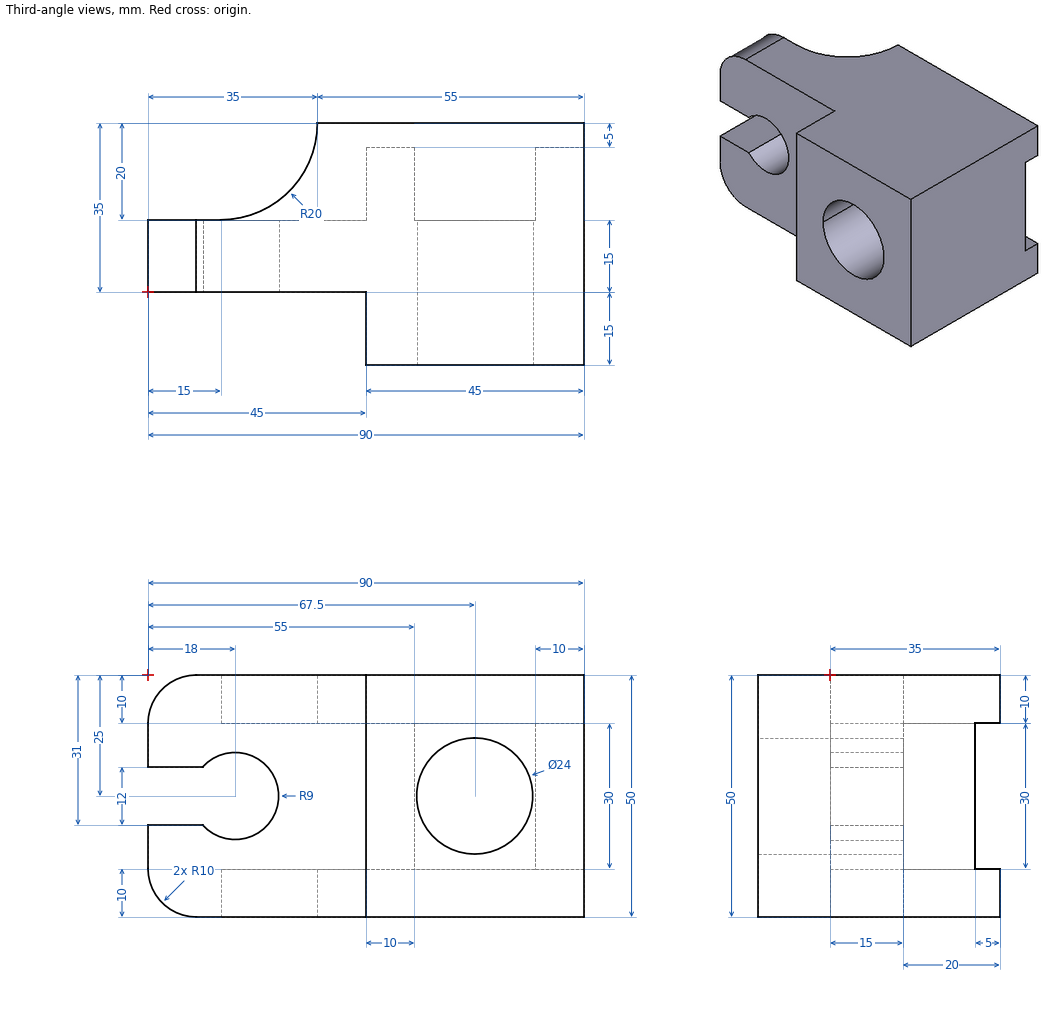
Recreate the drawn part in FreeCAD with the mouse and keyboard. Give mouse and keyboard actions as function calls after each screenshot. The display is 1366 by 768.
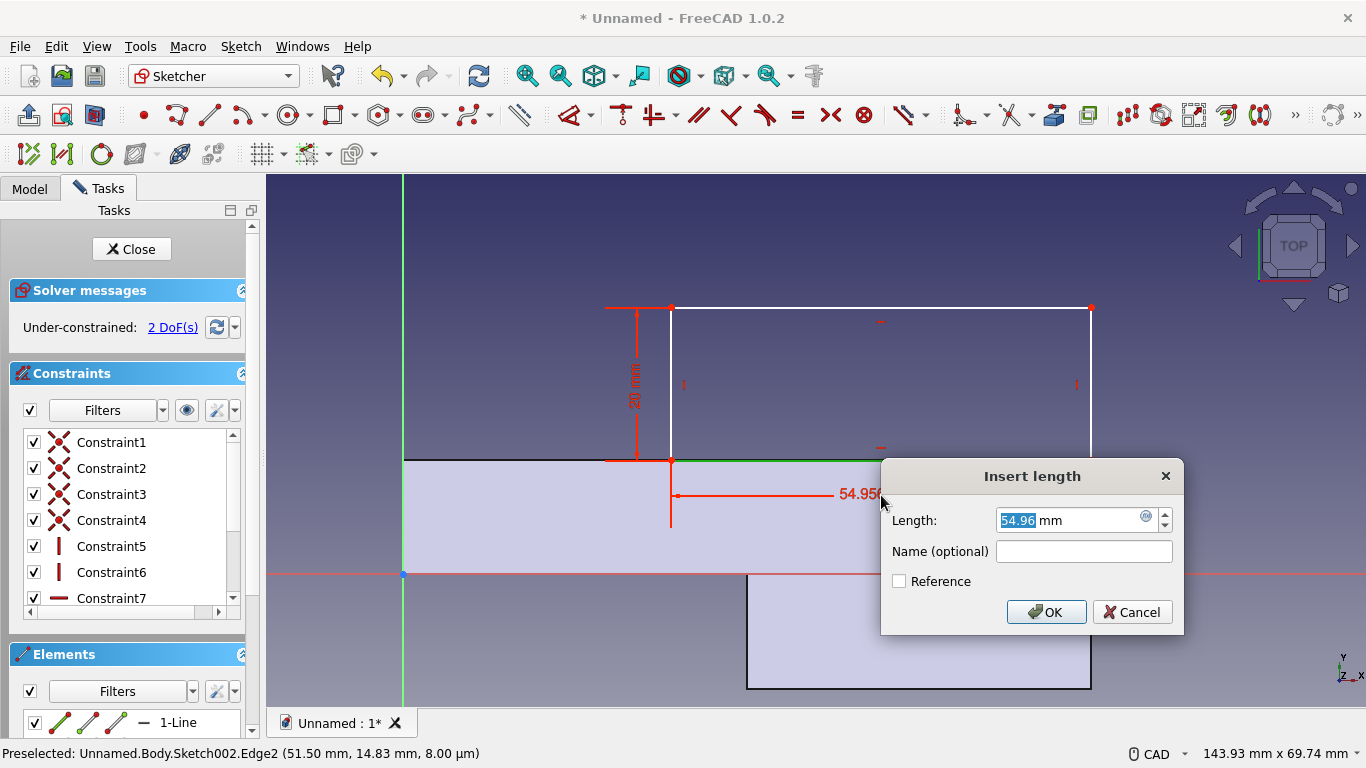
text(55)
key(Return)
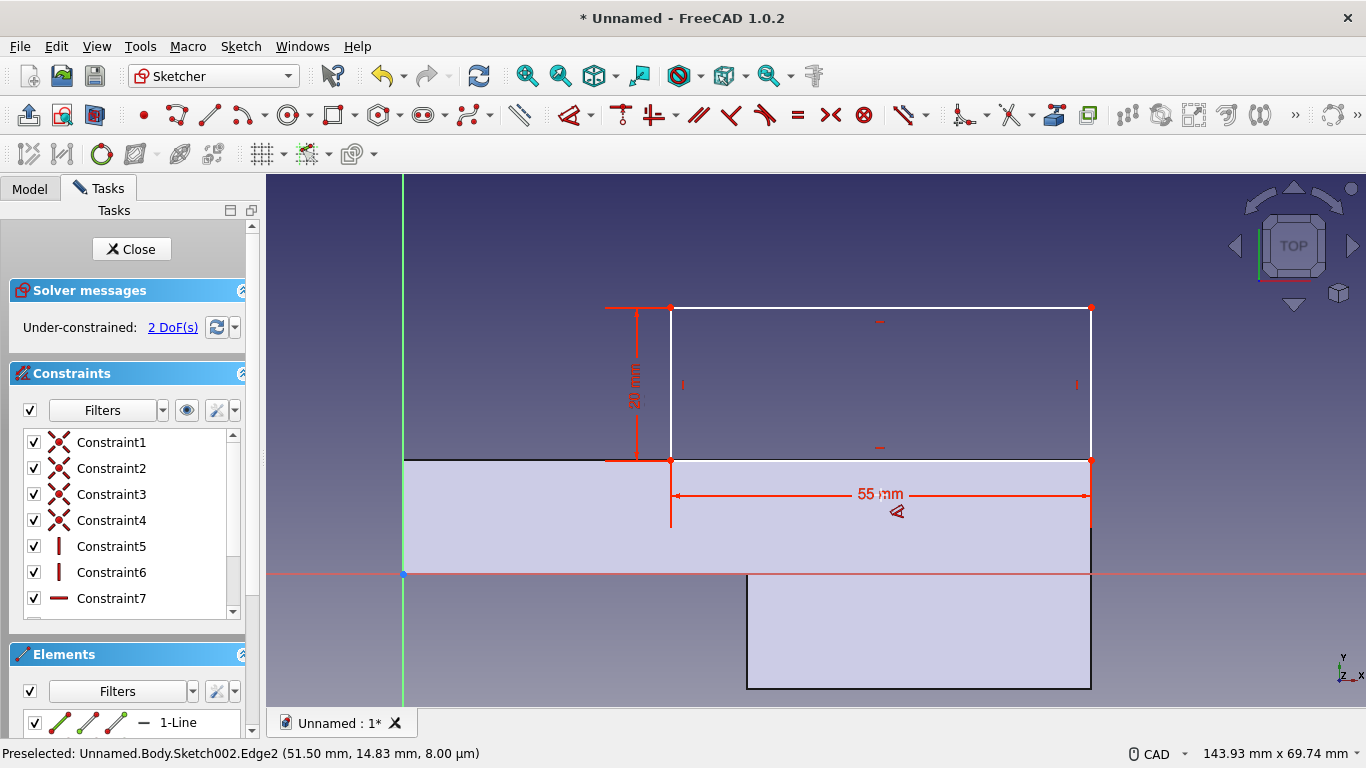
click(671, 308)
click(537, 608)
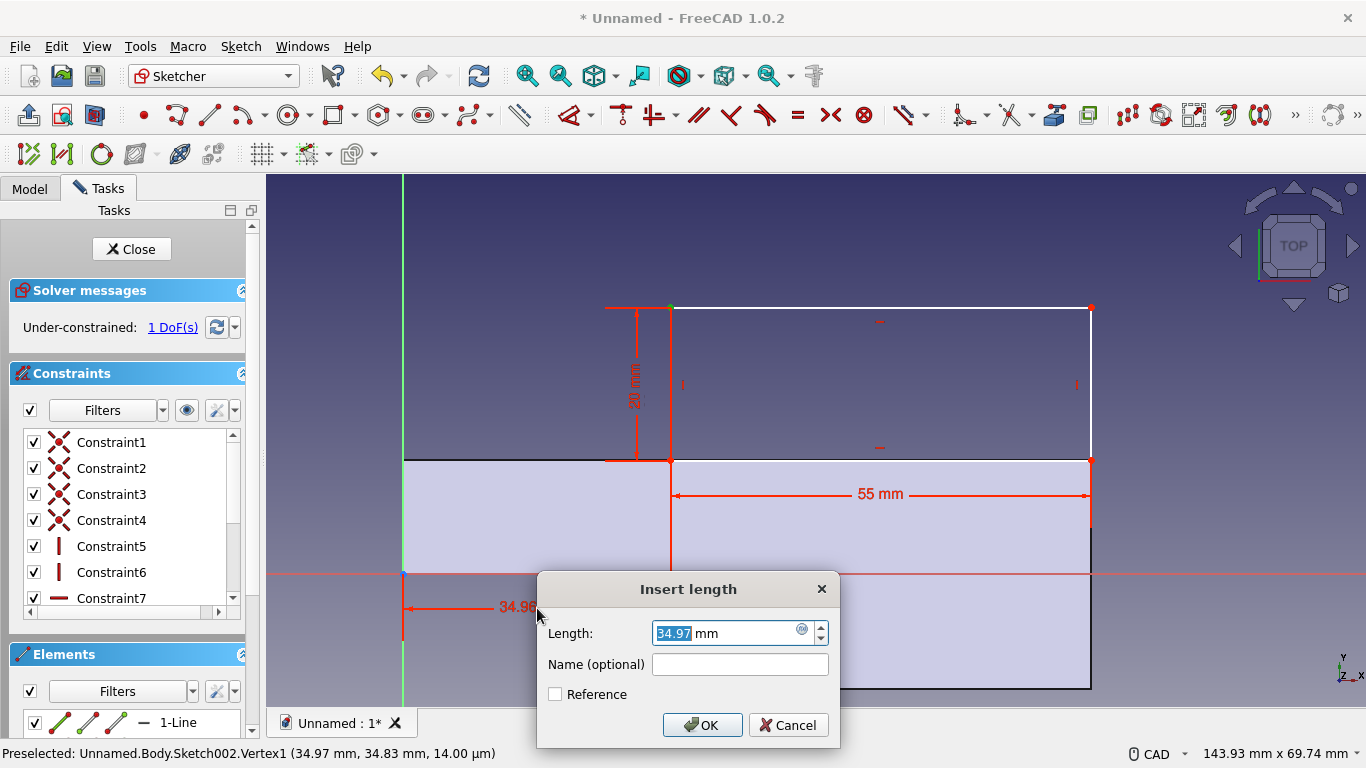
text(35)
key(Return)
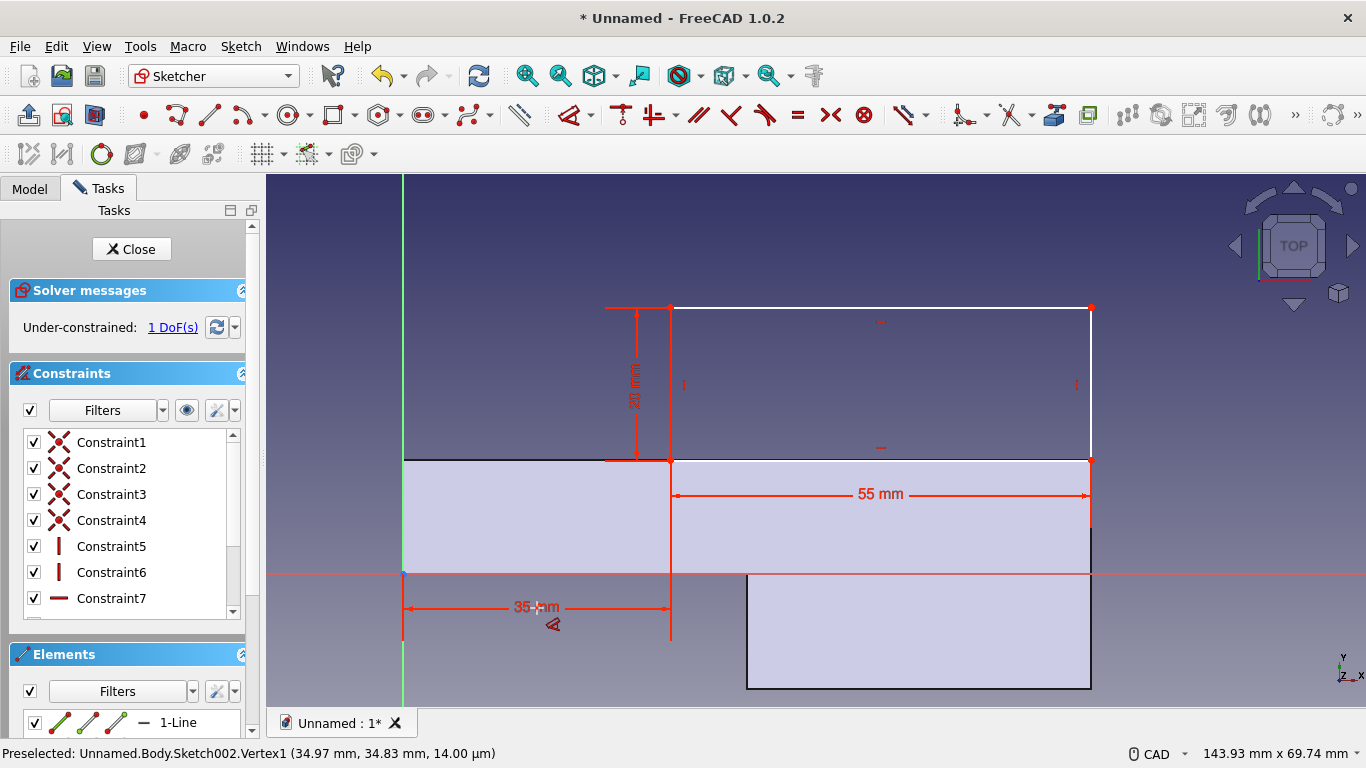
click(671, 308)
click(369, 441)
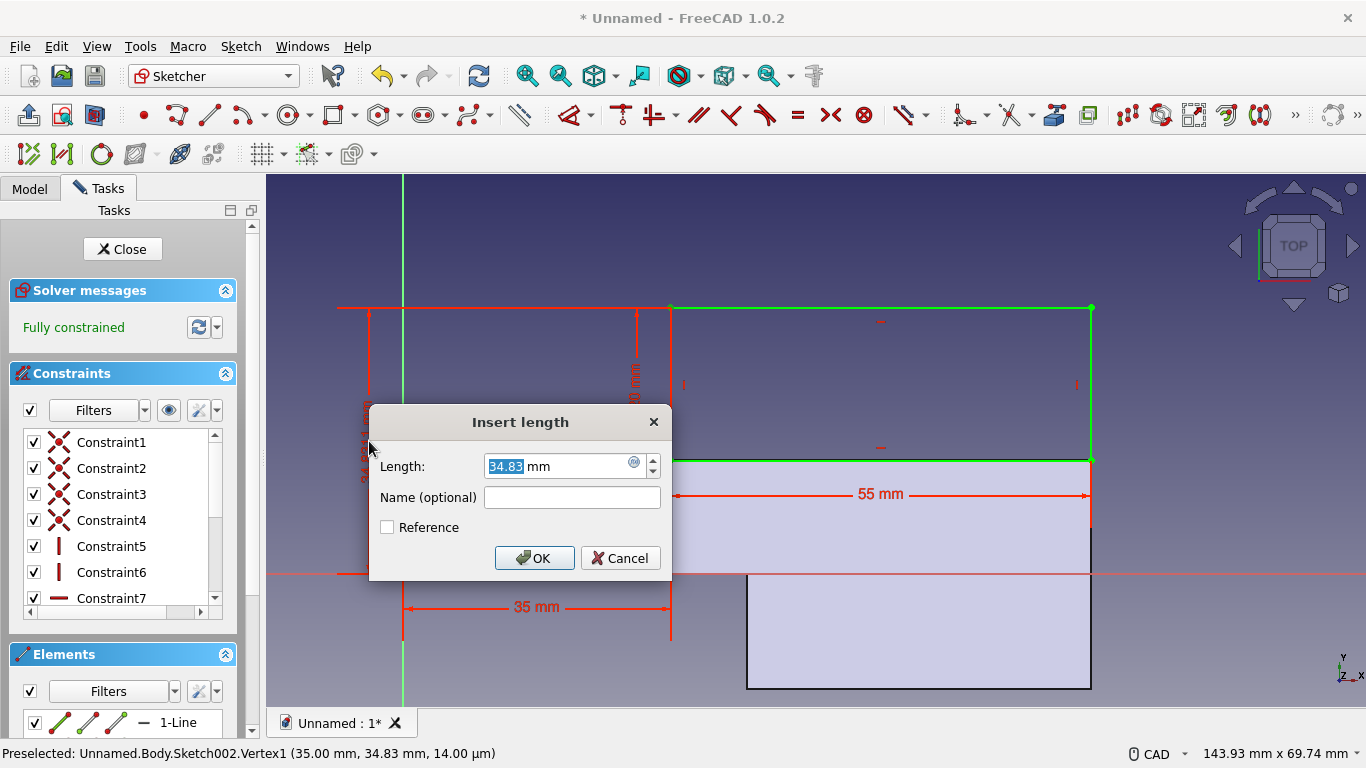
text(35)
key(Return)
key(Escape)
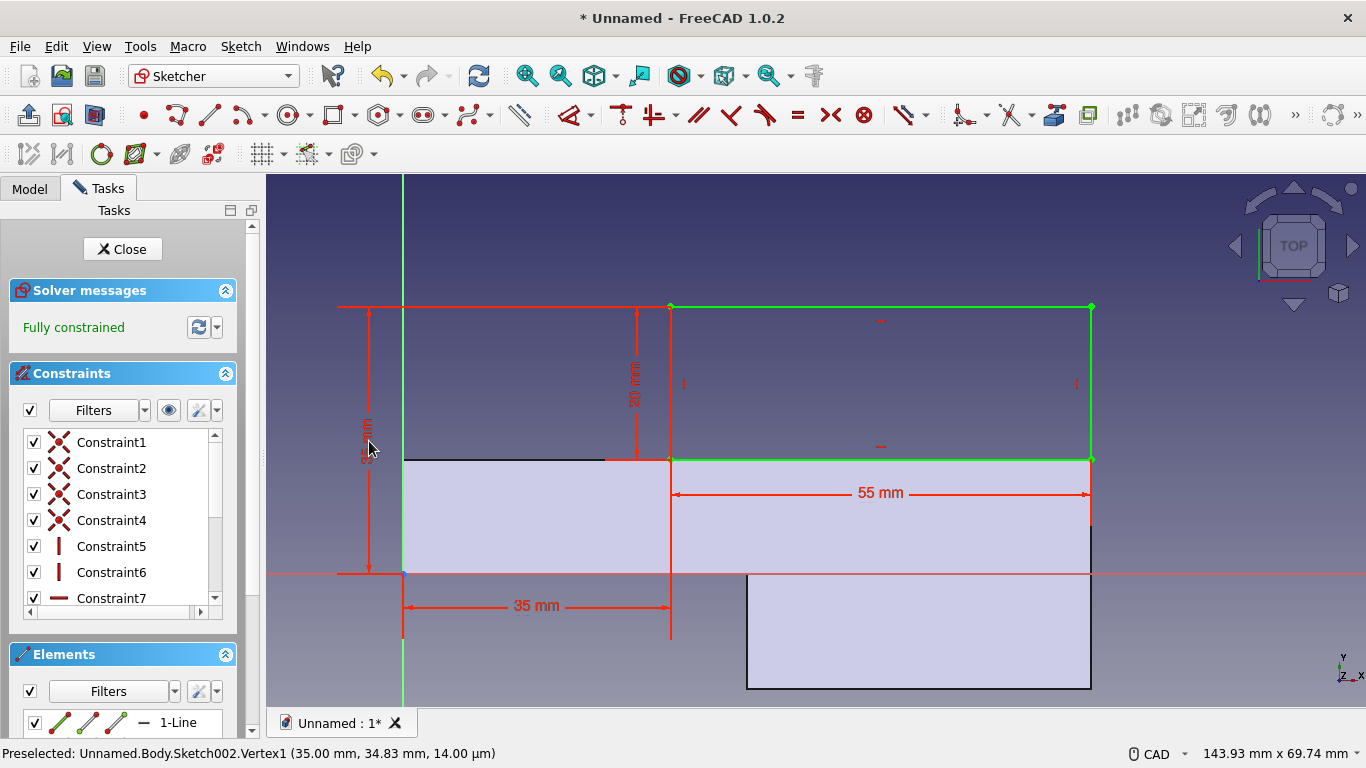
click(123, 249)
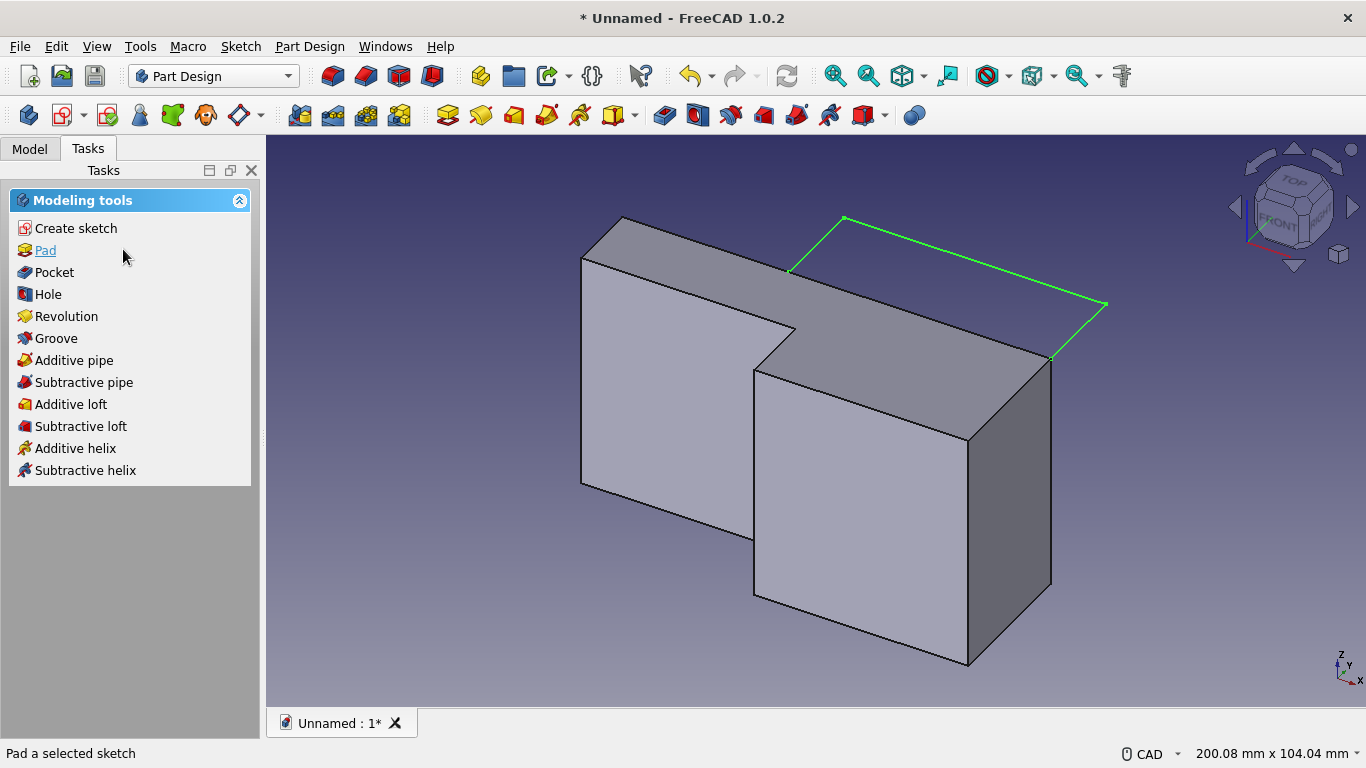
click(448, 116)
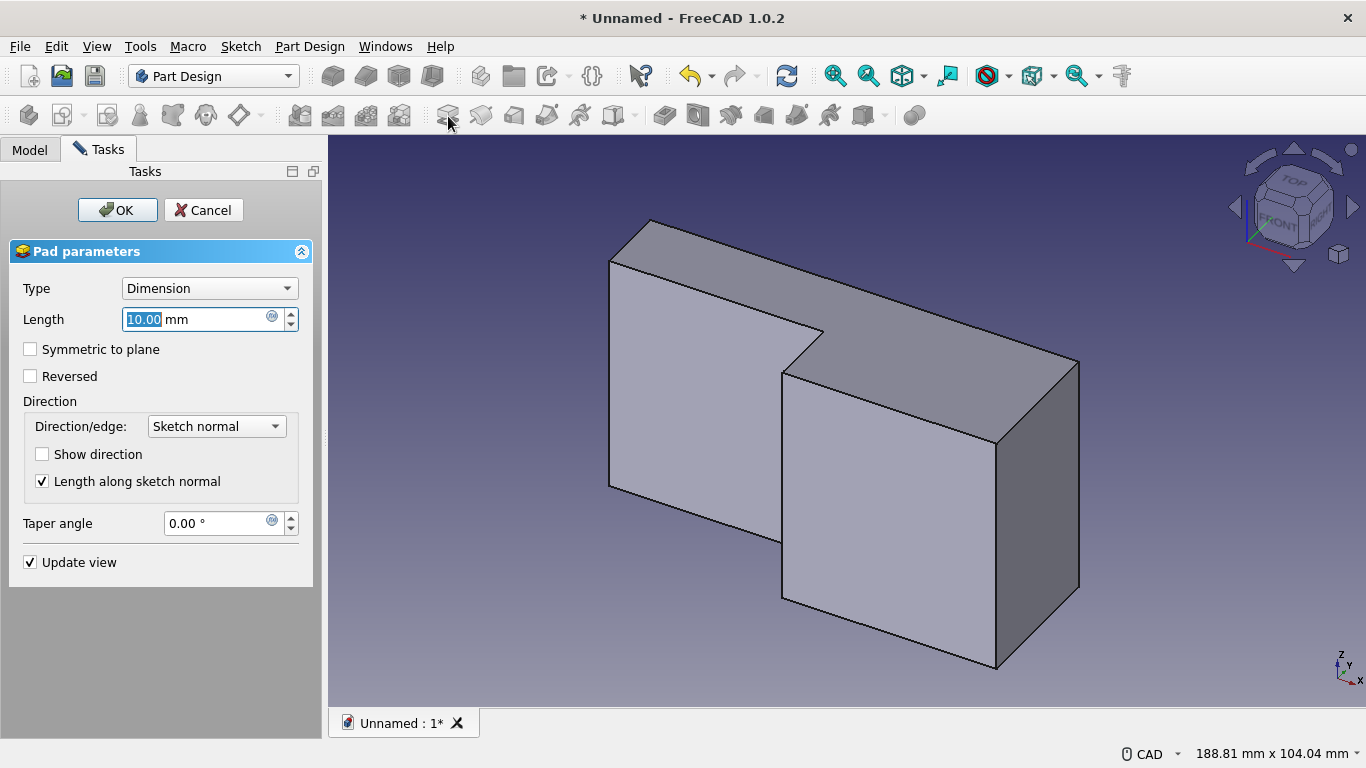
text(50)
key(Tab)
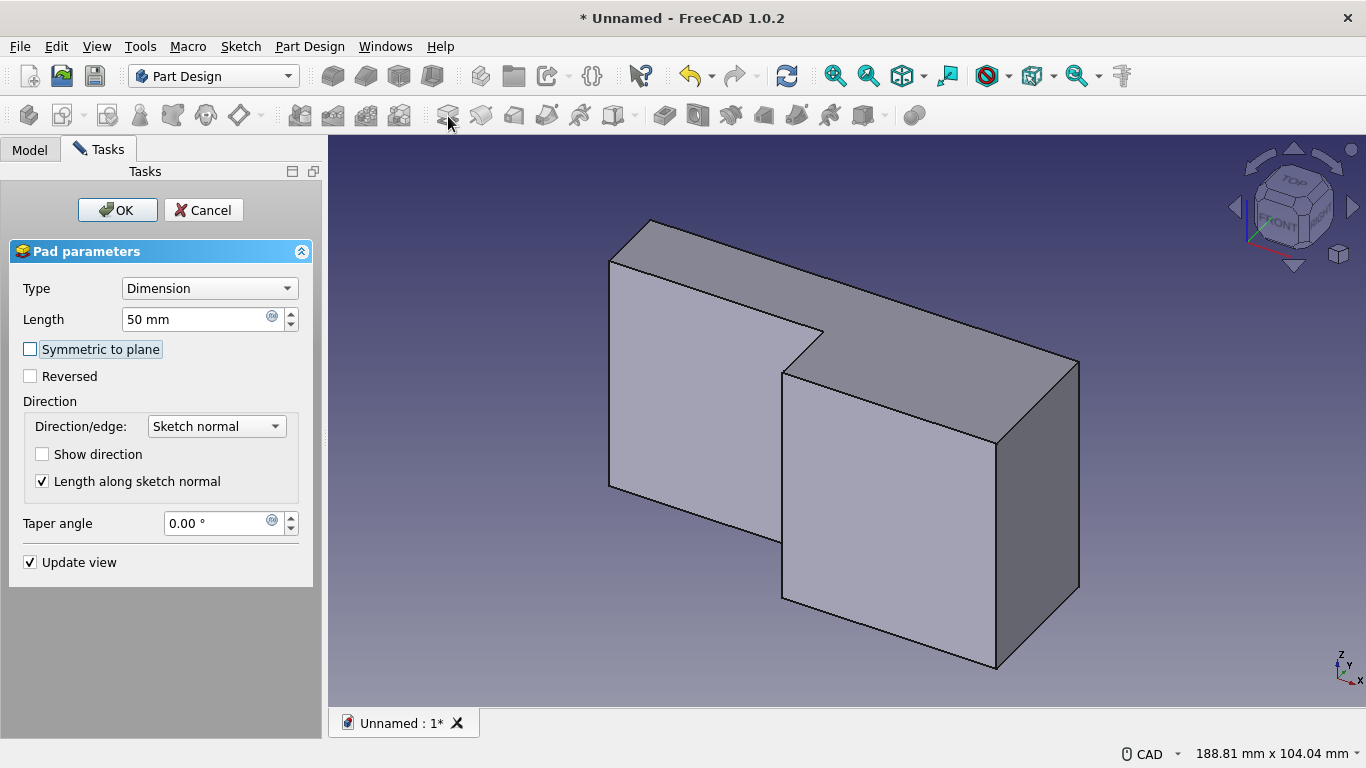
click(31, 376)